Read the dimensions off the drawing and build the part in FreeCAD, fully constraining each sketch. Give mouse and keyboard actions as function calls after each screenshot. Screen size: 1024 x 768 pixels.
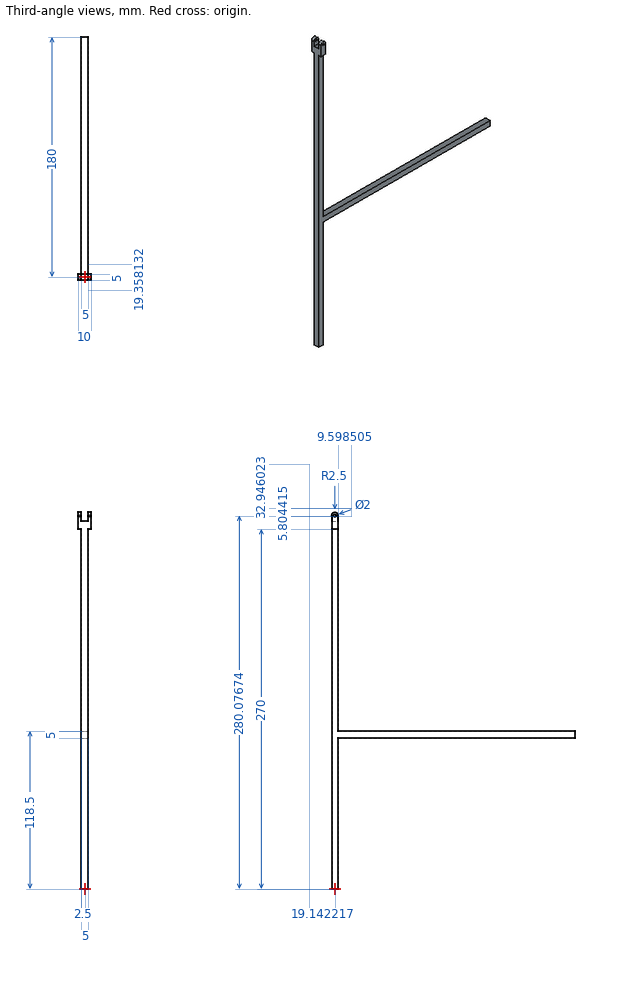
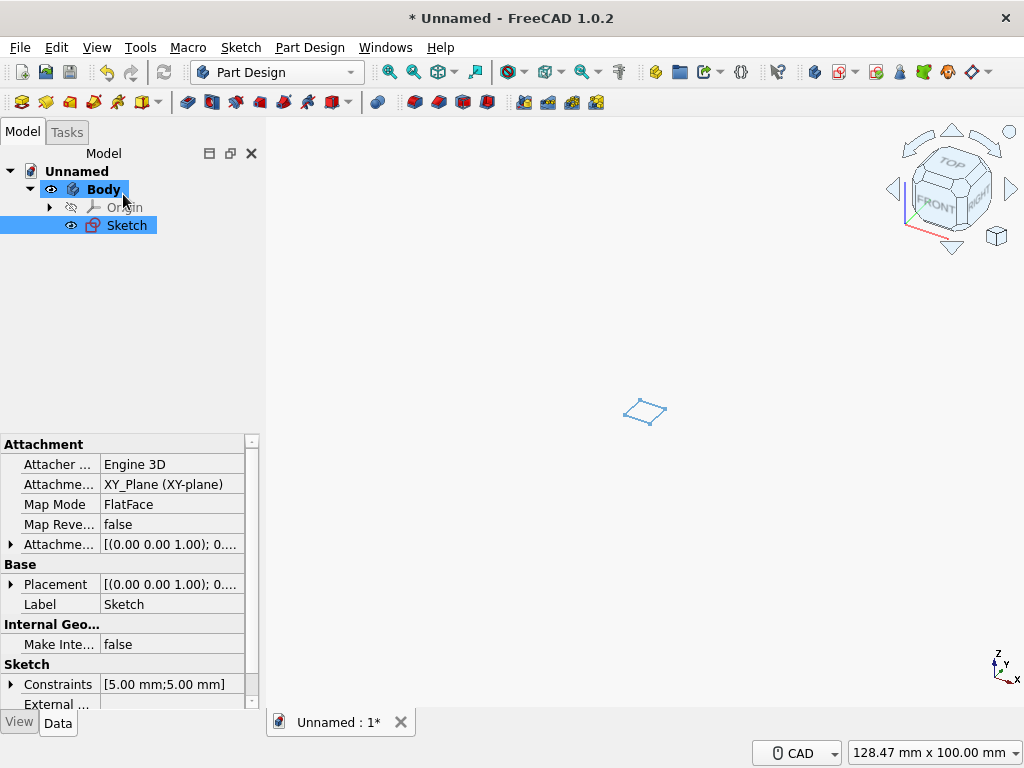
click(22, 102)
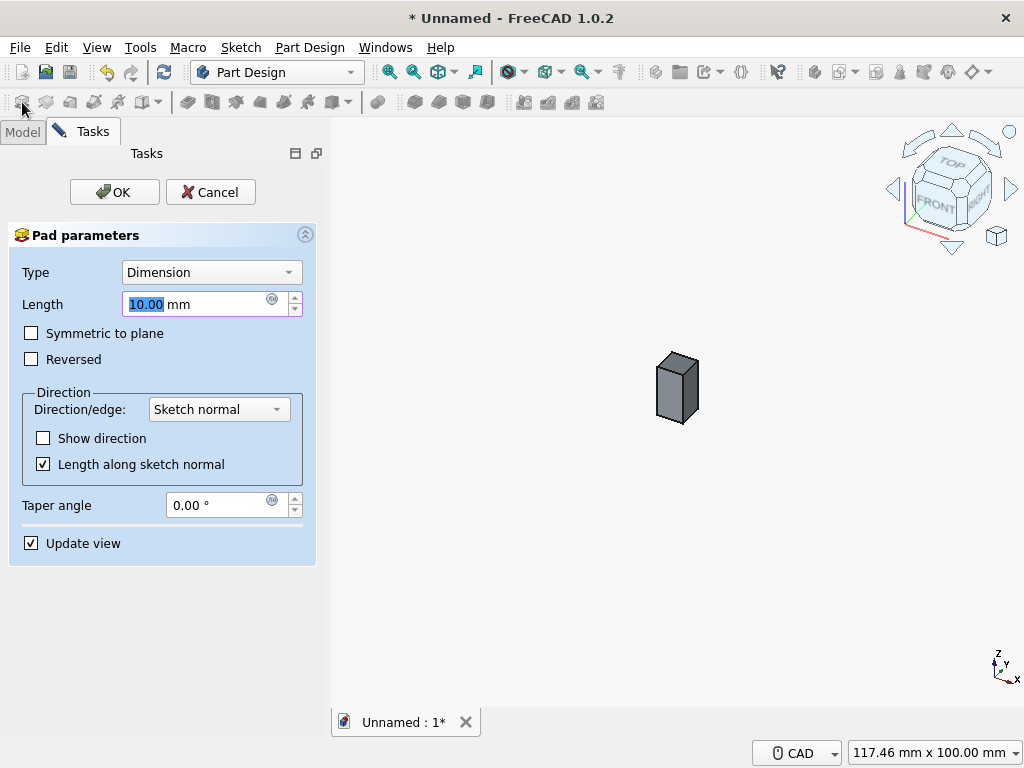
text(270)
key(Tab)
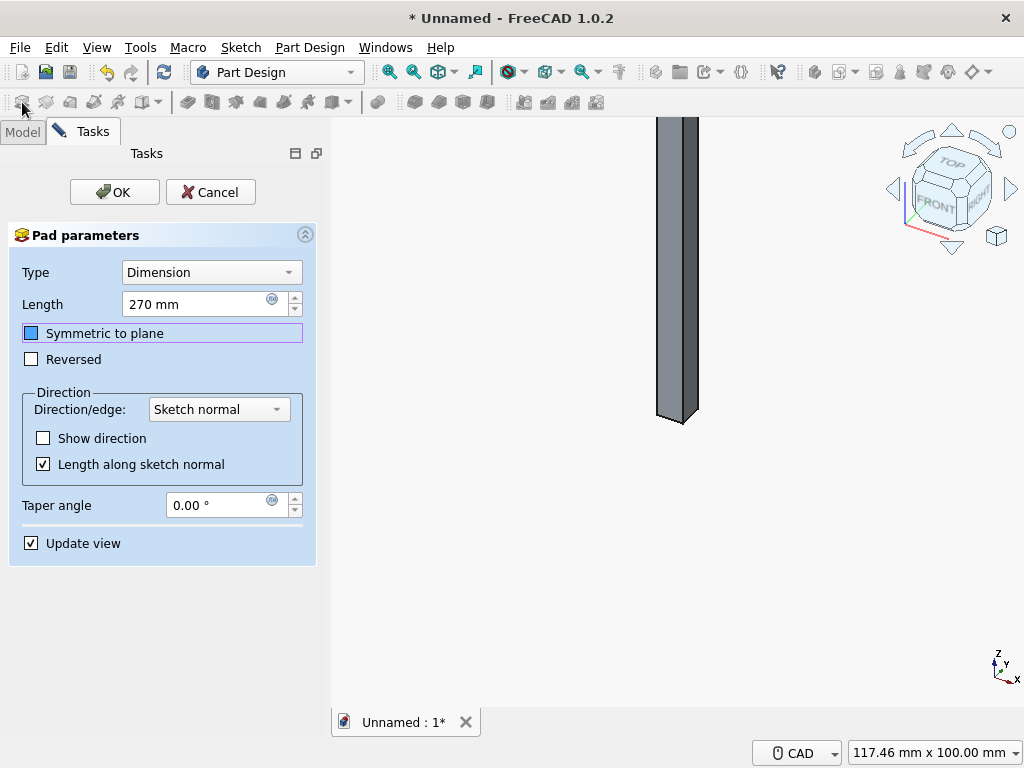
click(115, 192)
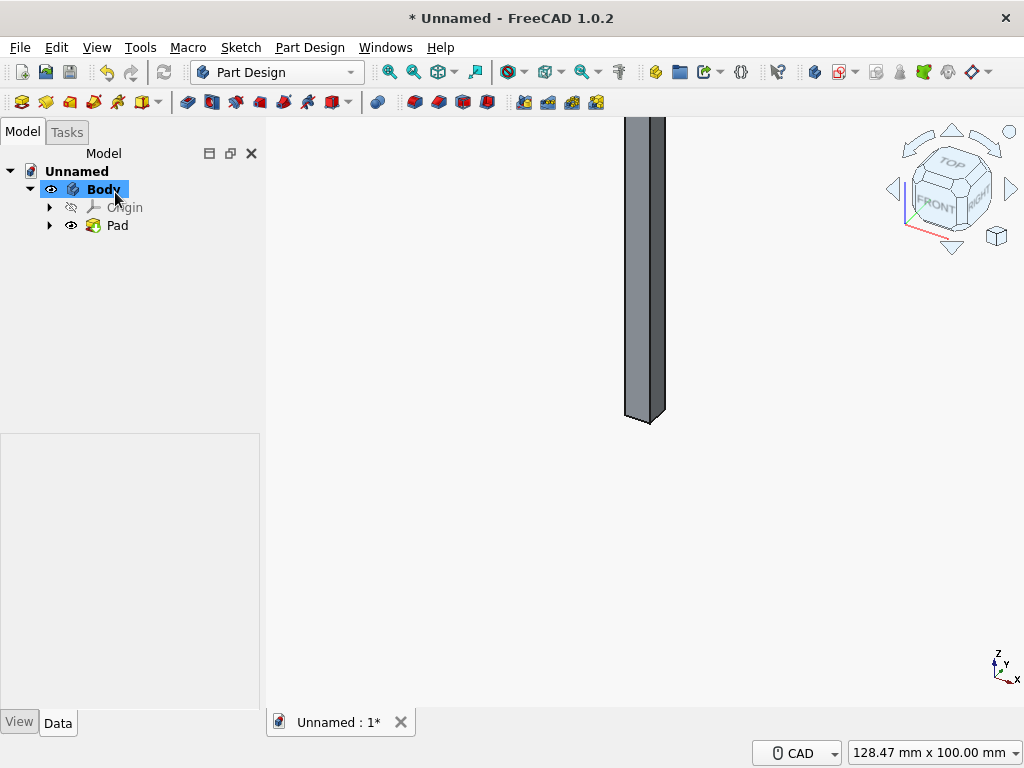
click(390, 72)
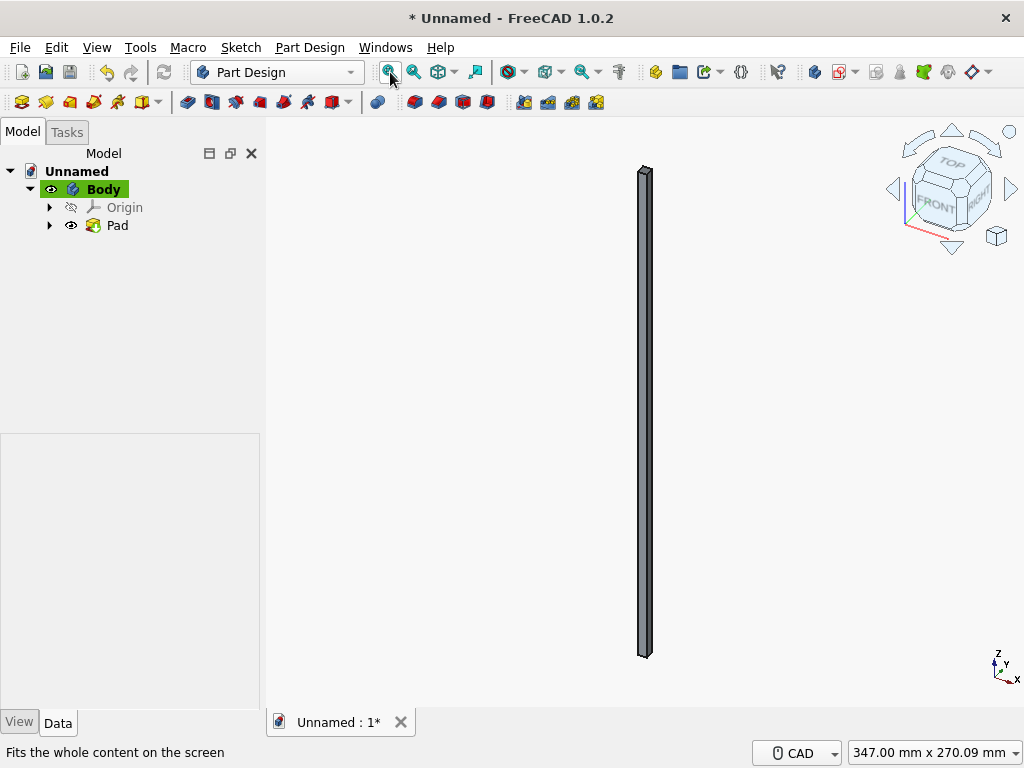
scroll(645, 169, up, 4)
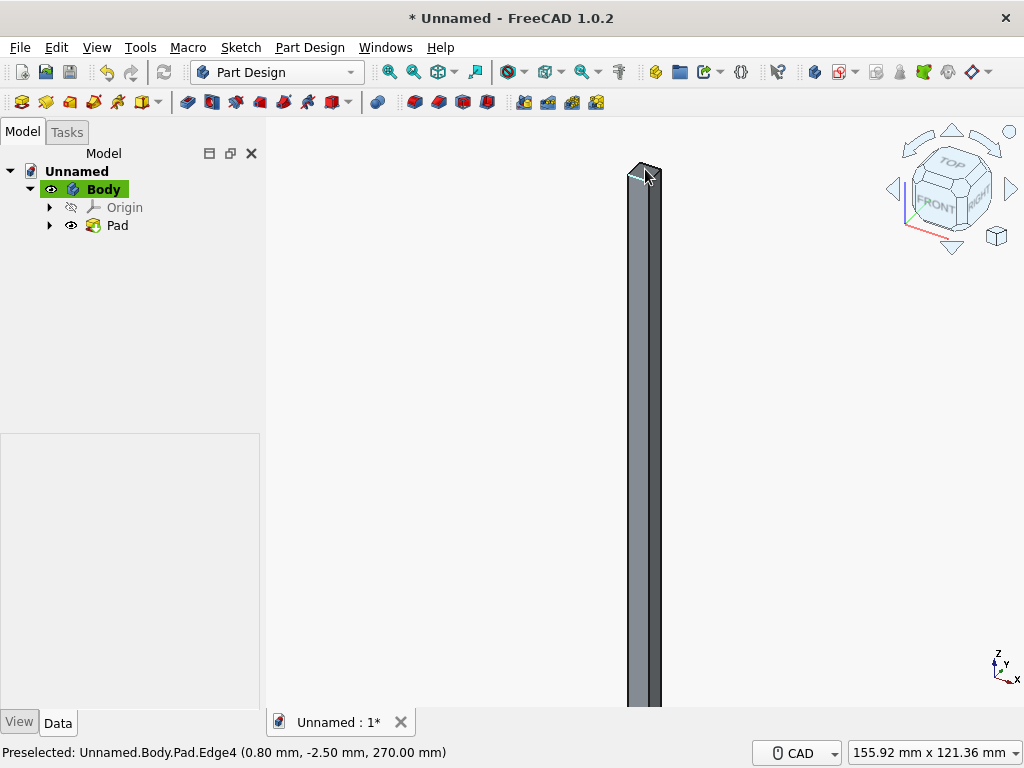
click(646, 169)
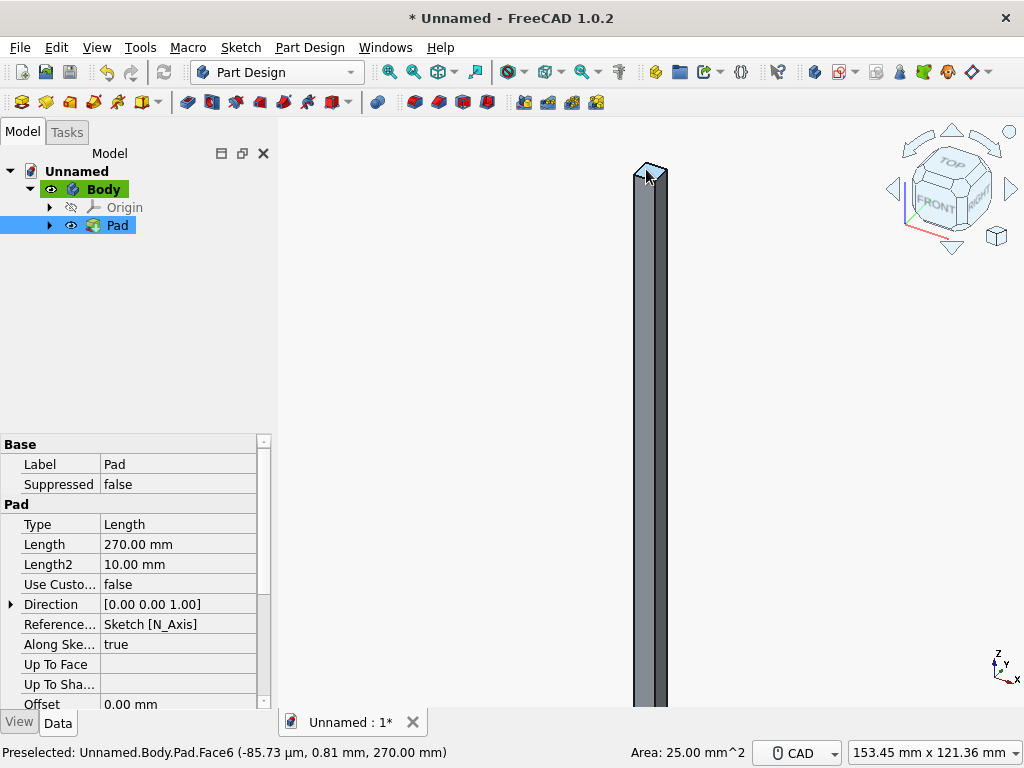
click(840, 72)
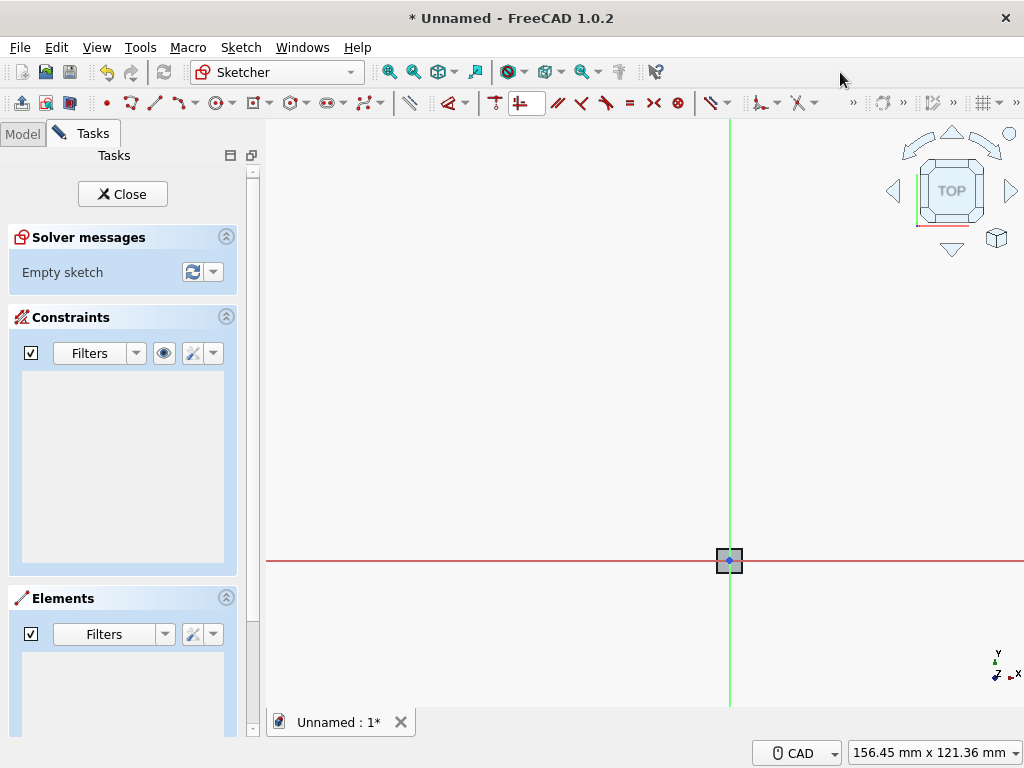
scroll(749, 579, up, 11)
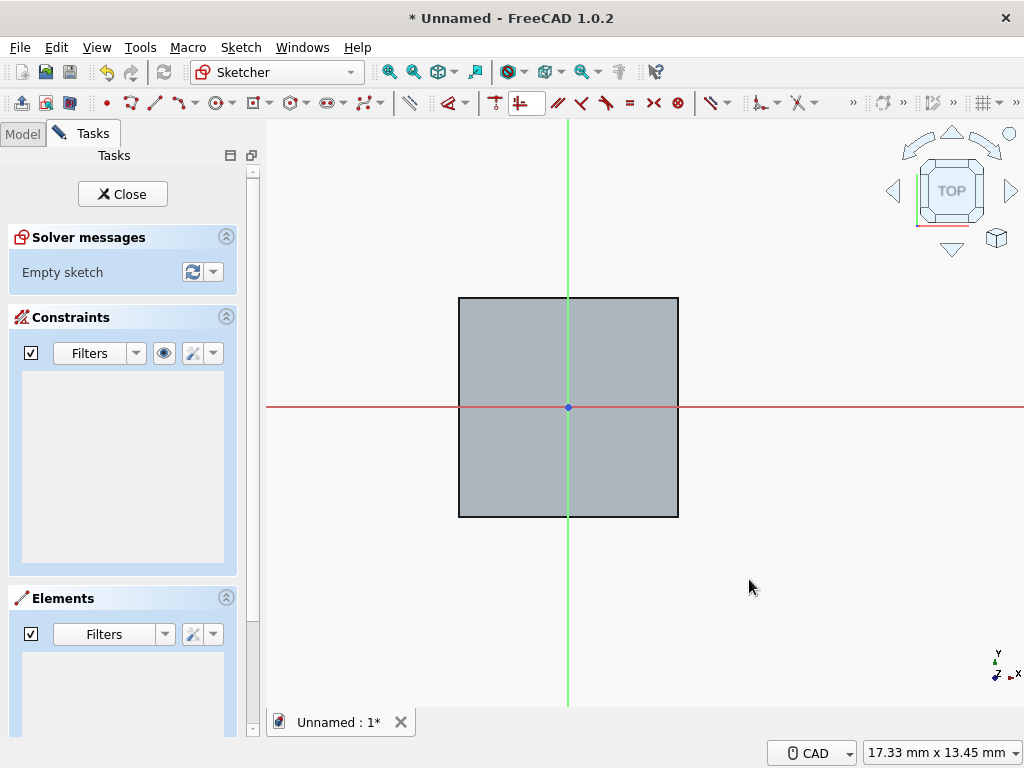
click(254, 104)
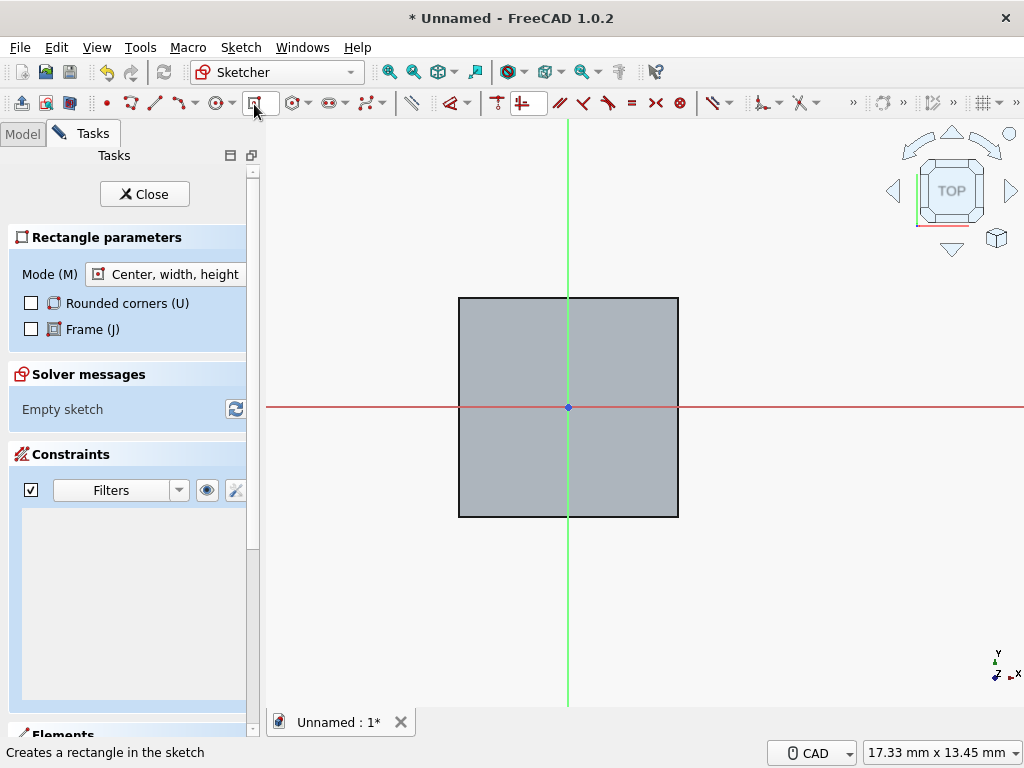
click(568, 407)
click(787, 298)
key(Escape)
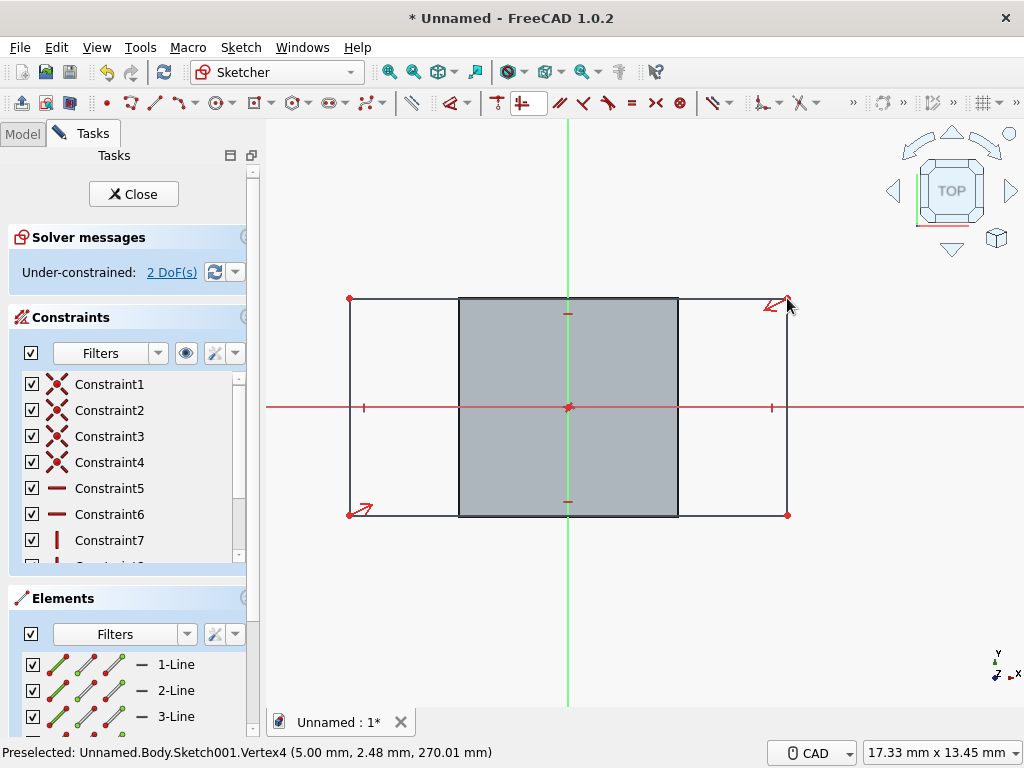
click(450, 104)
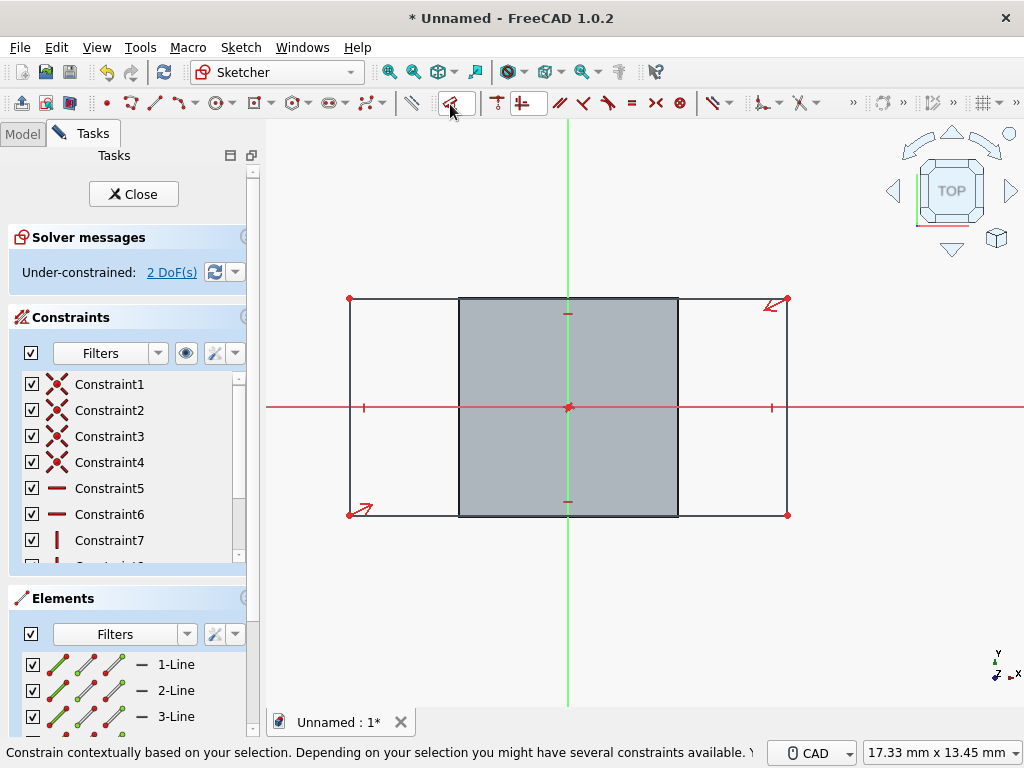
click(787, 451)
click(821, 358)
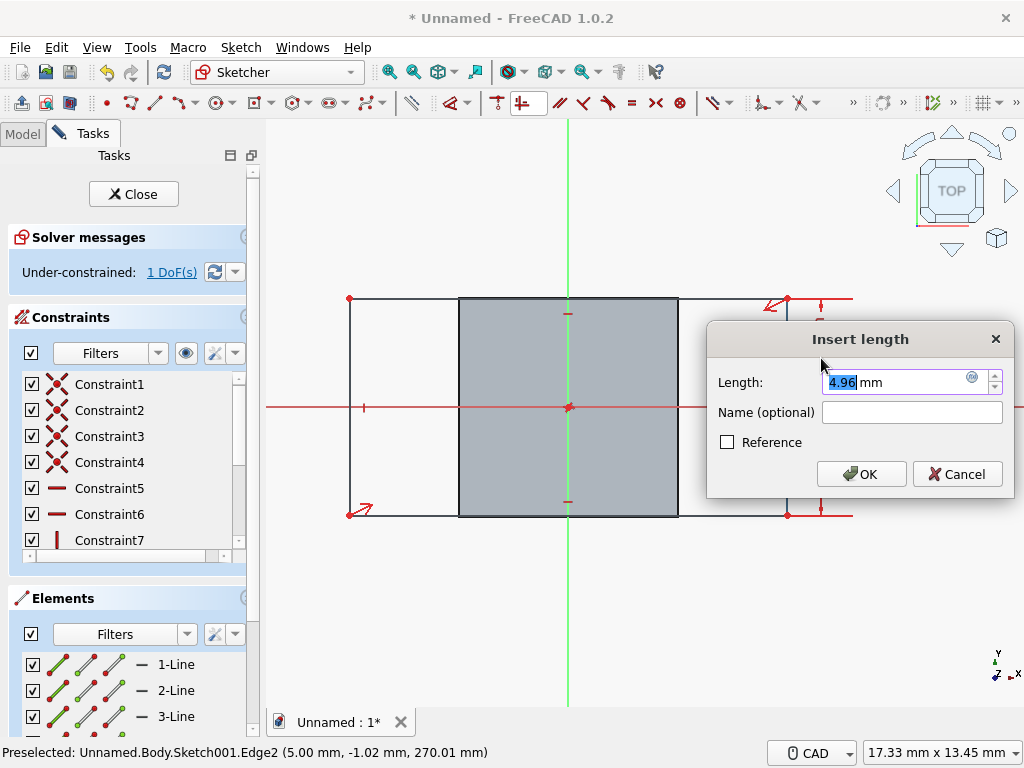
text(5)
key(Return)